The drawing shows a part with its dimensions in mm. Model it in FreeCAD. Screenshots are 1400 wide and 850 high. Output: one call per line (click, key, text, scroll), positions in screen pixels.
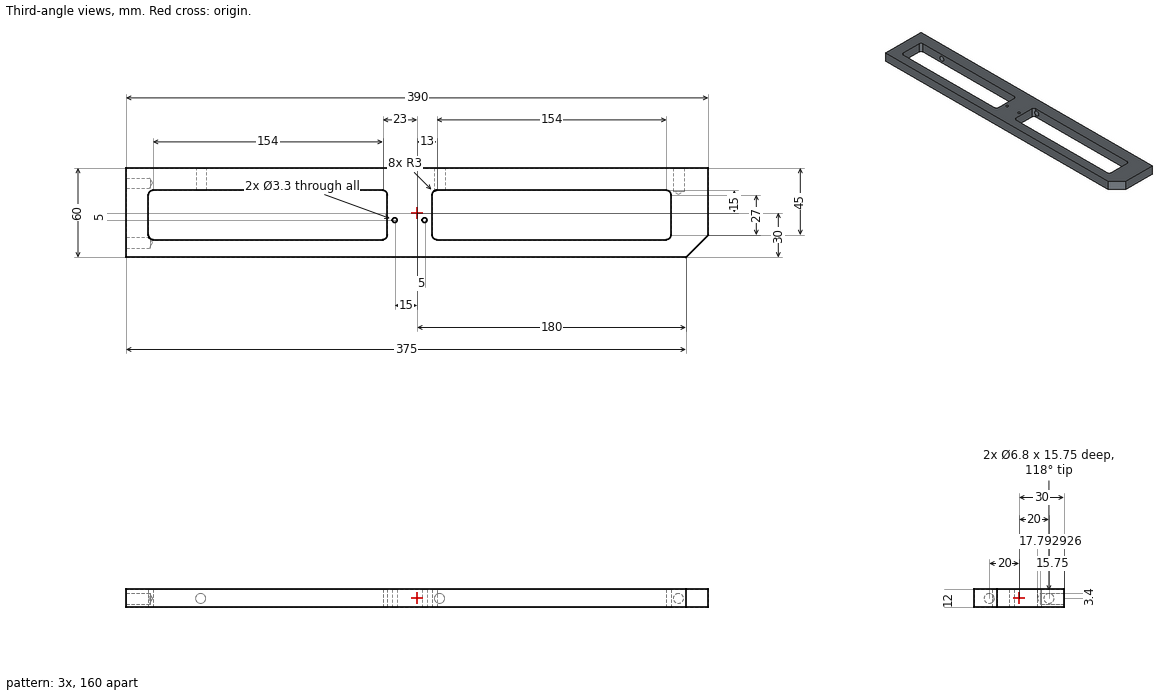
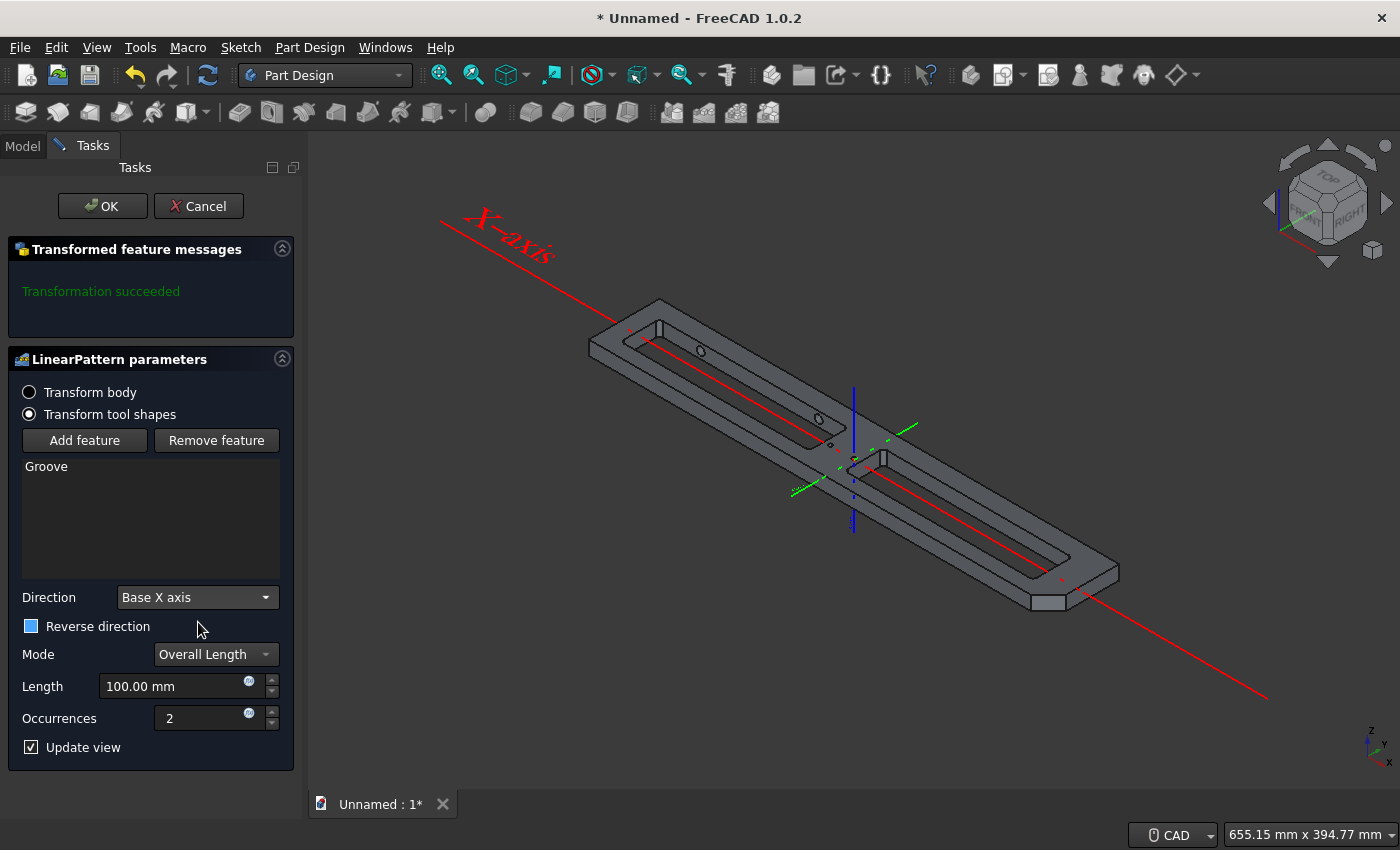
click(217, 654)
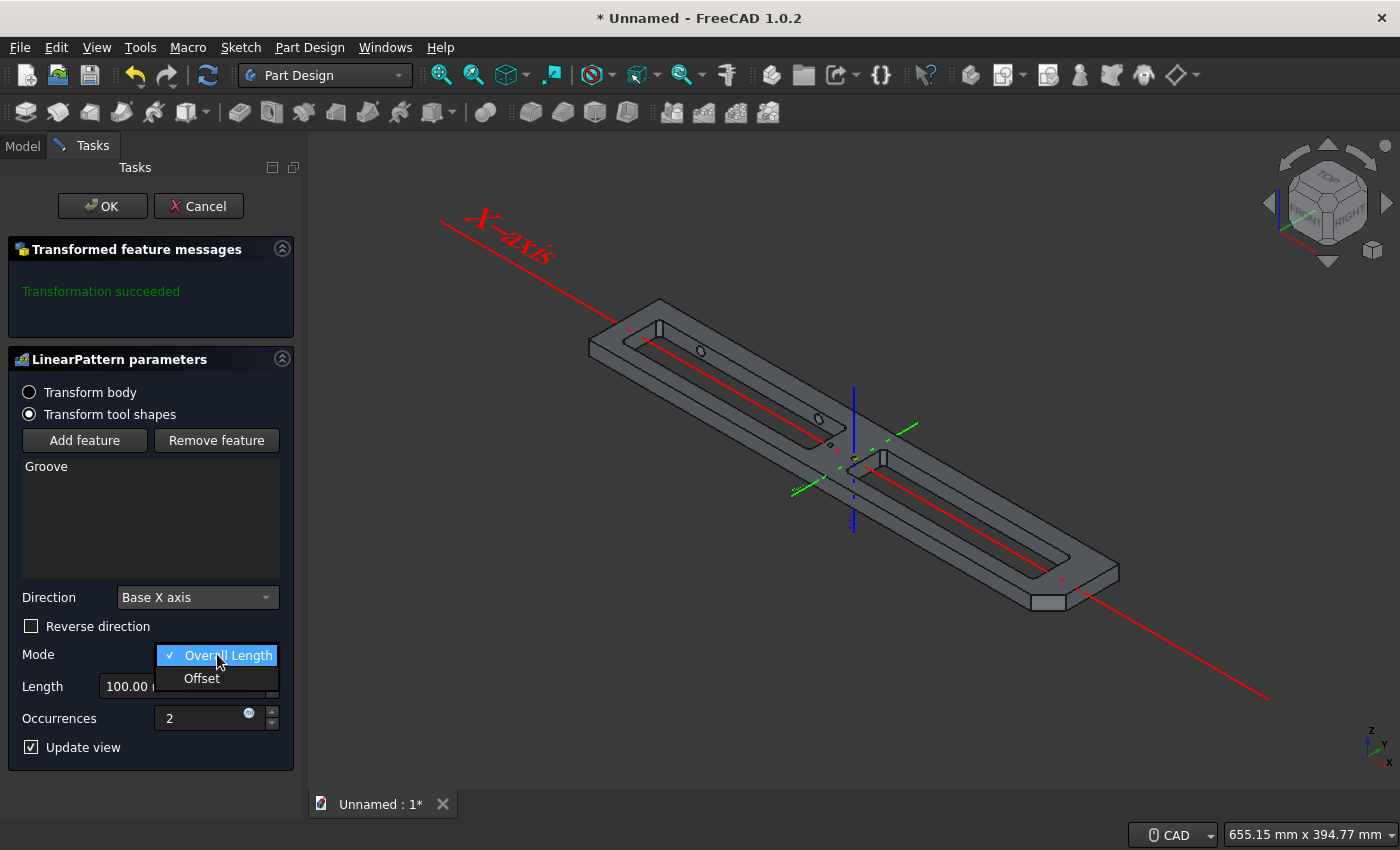
click(216, 678)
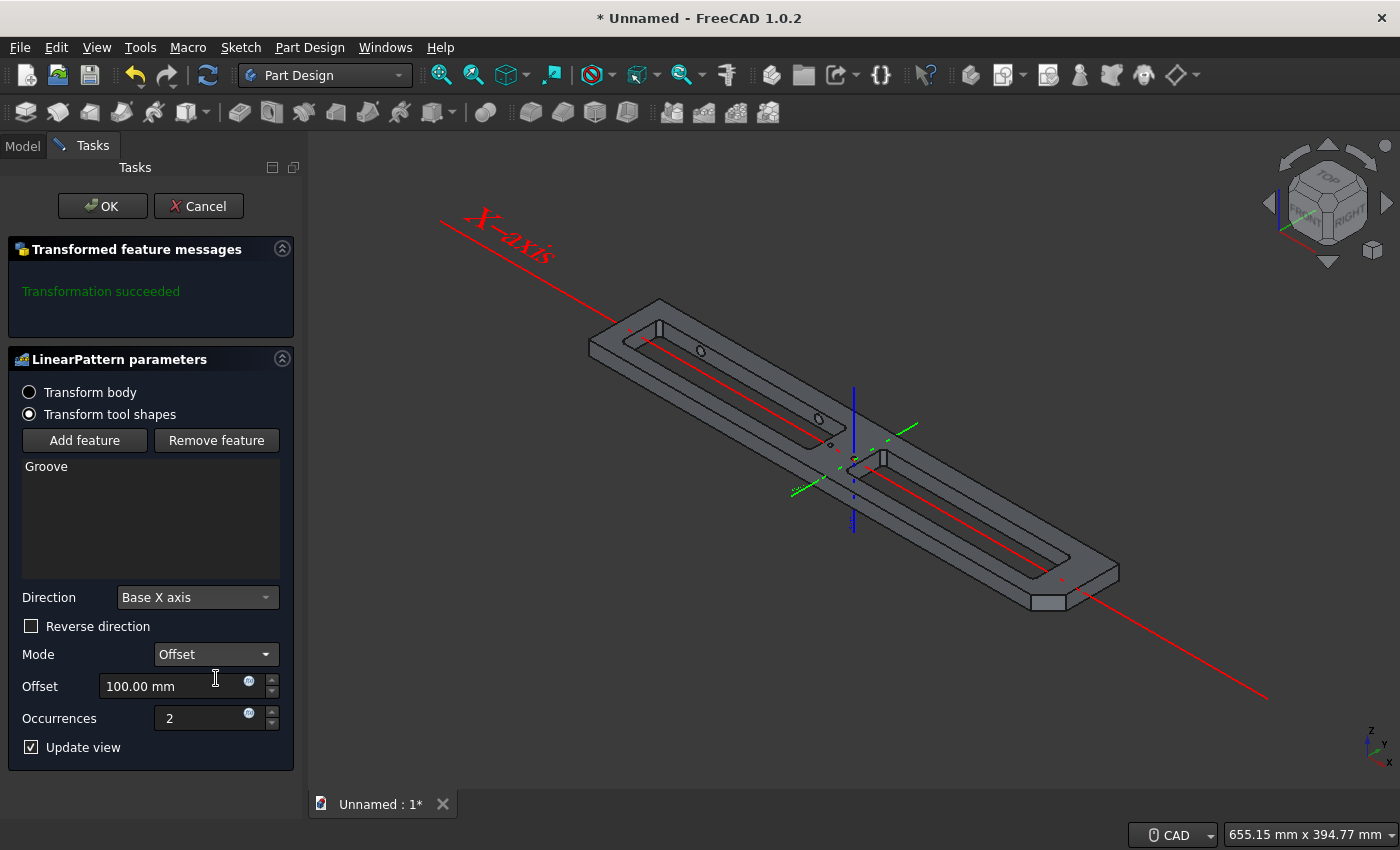
triple_click(182, 686)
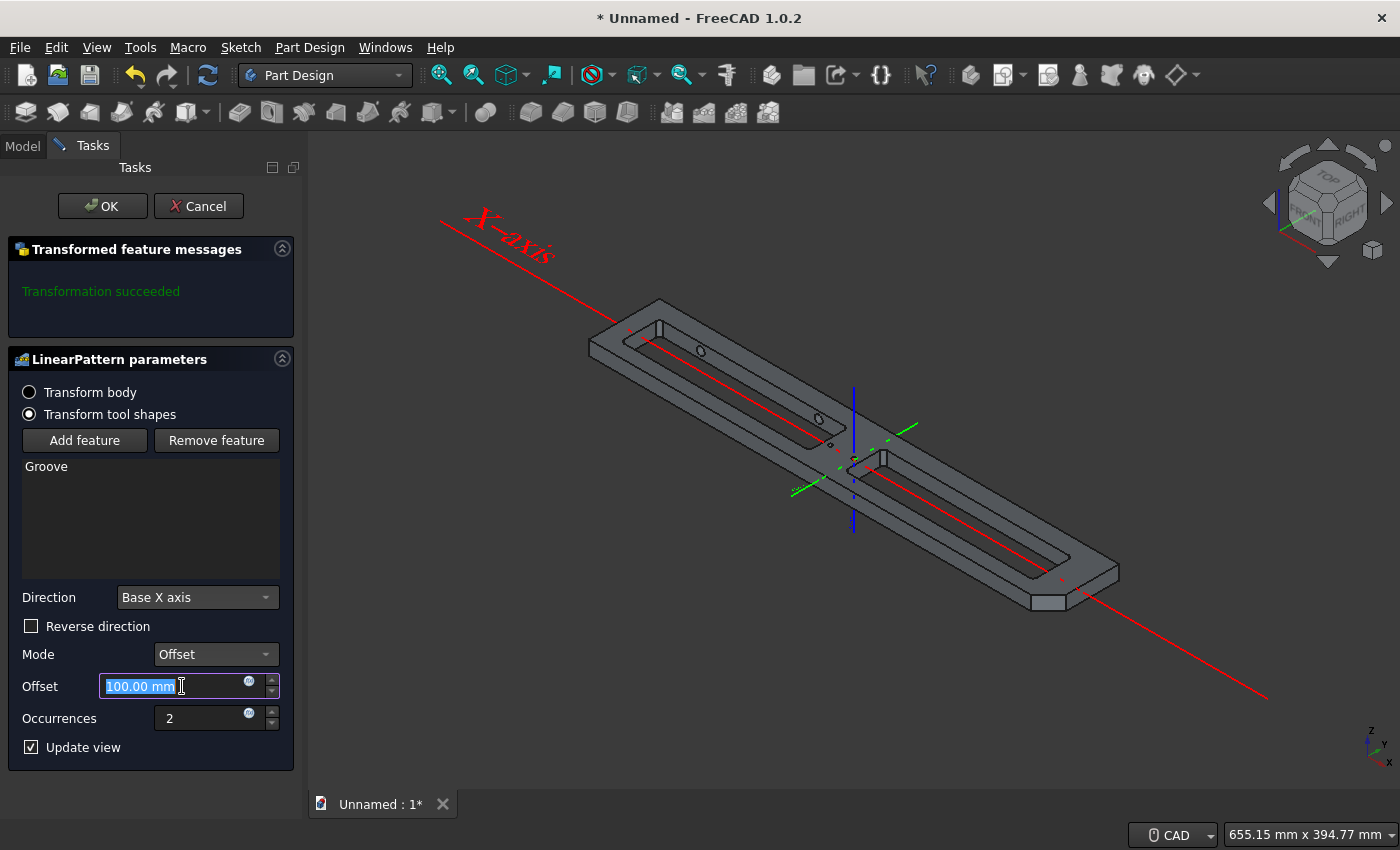
text(160)
key(Tab)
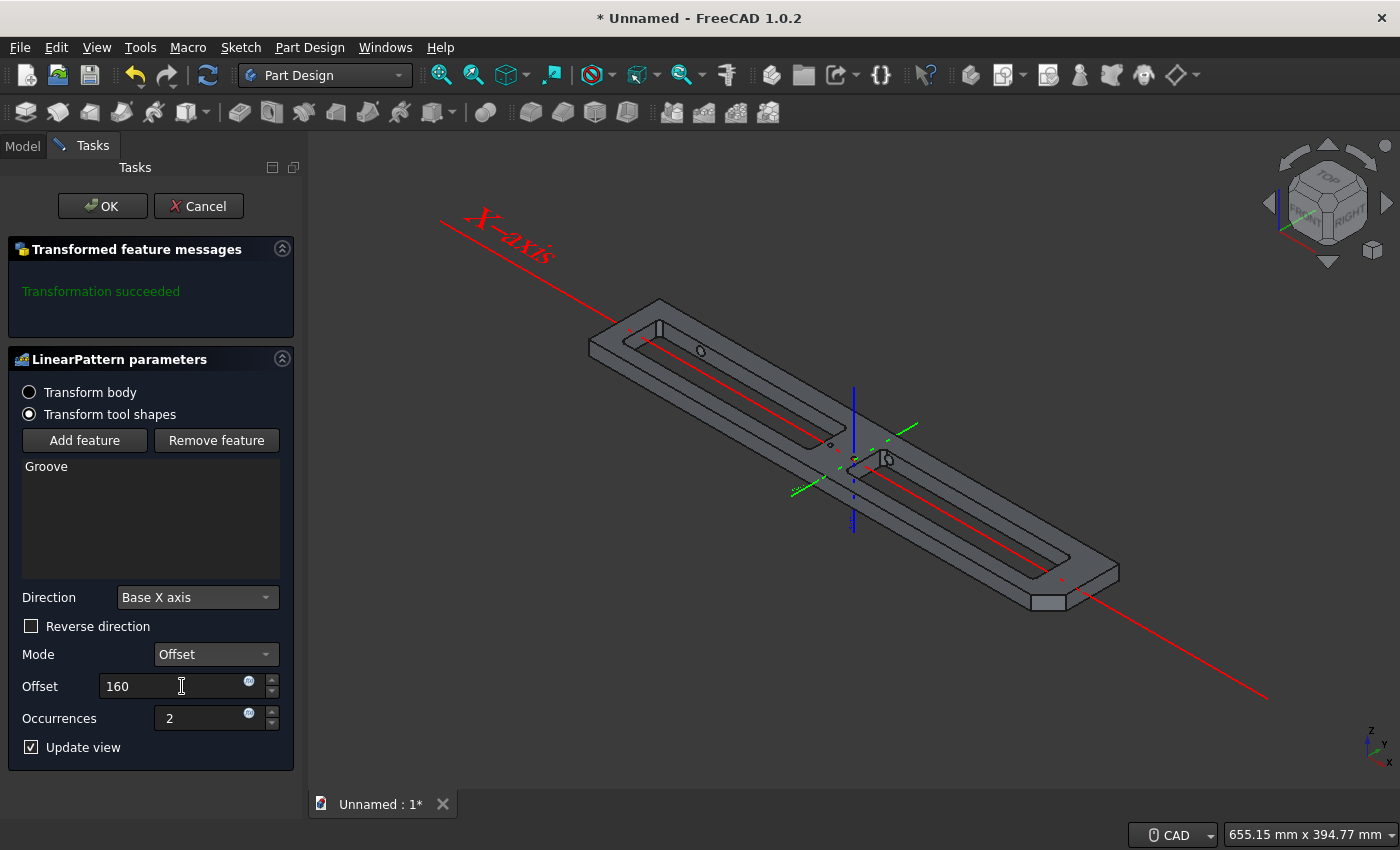
triple_click(209, 718)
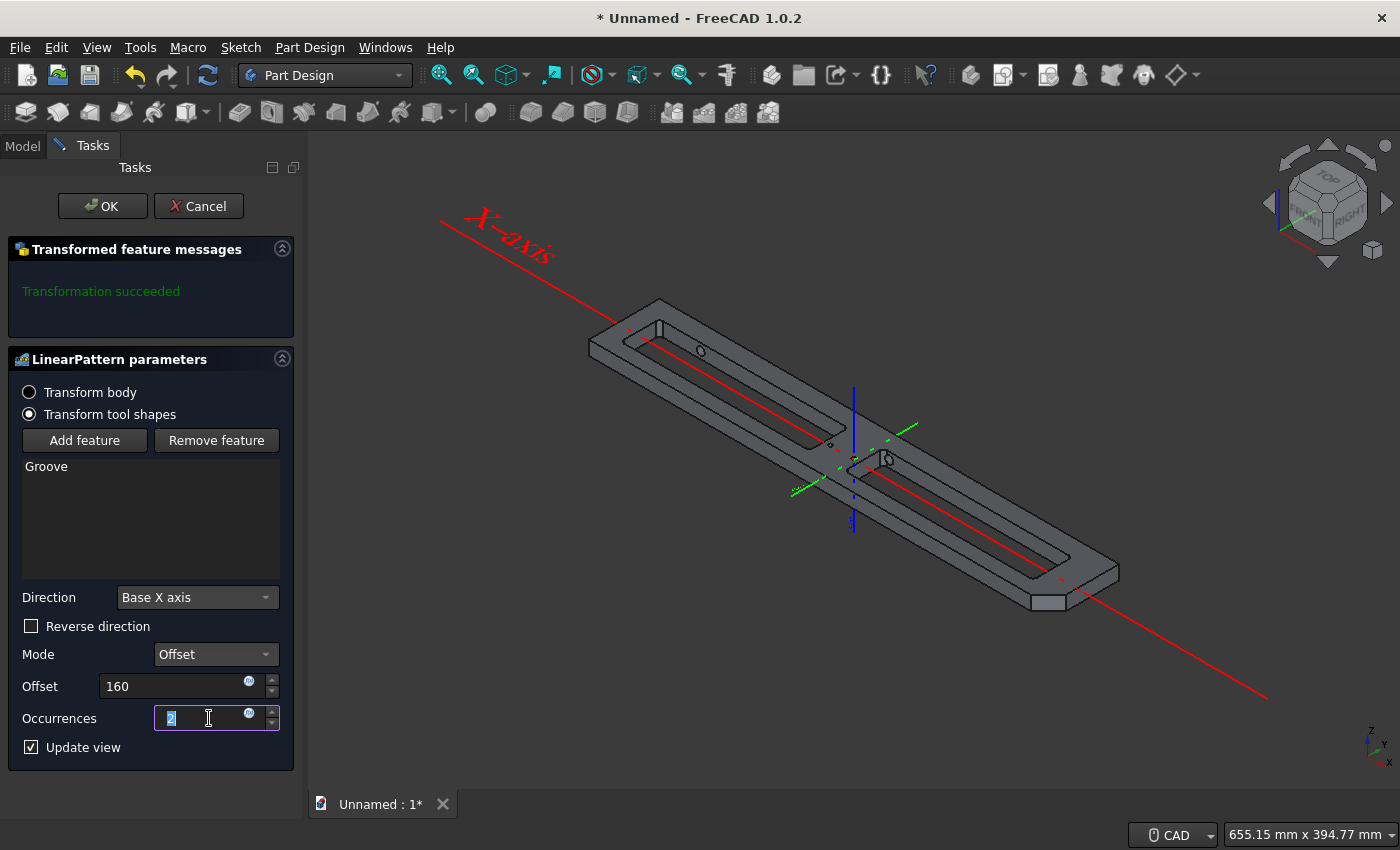
text(3)
key(Tab)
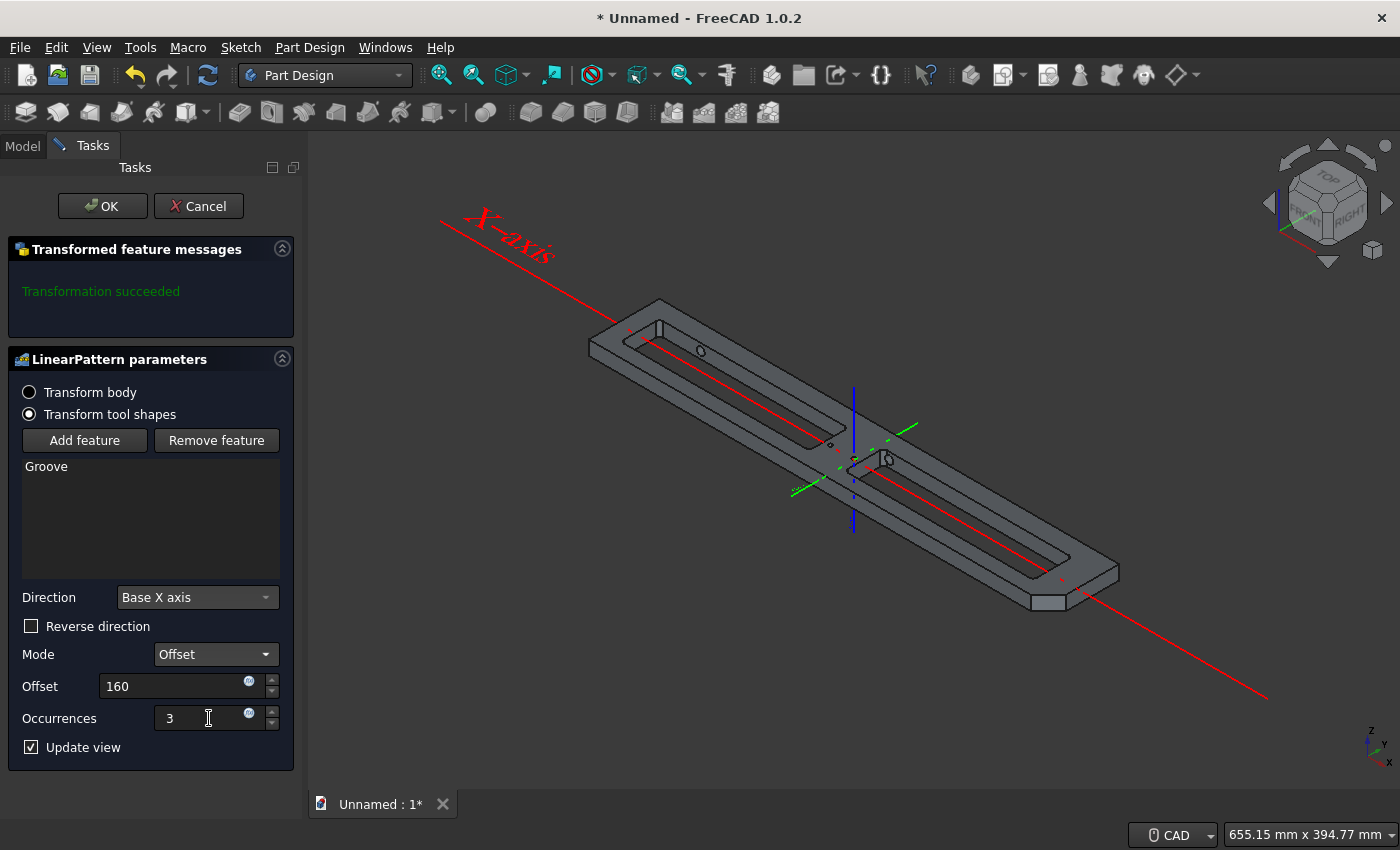
click(103, 206)